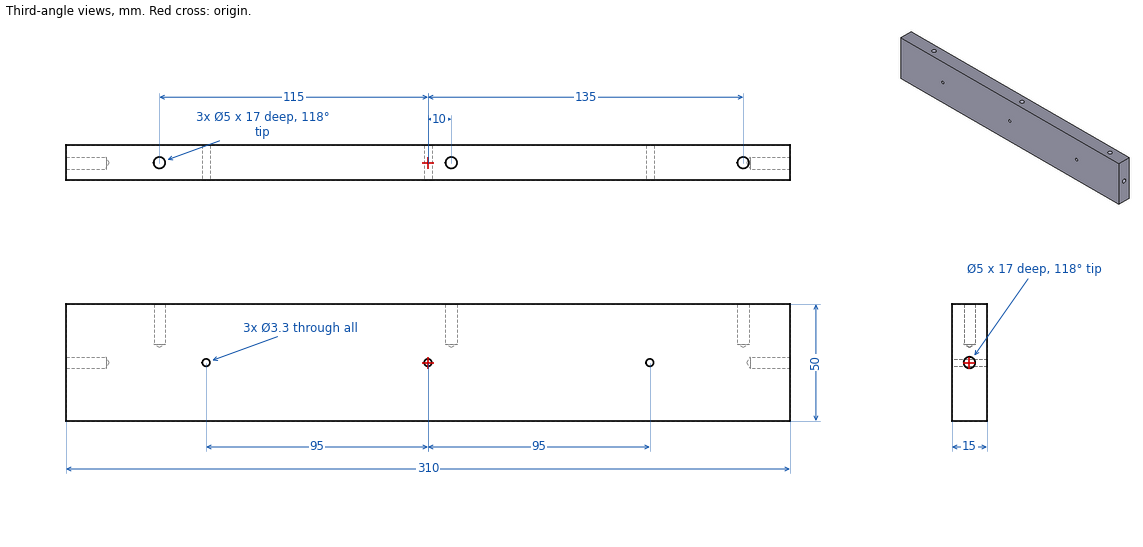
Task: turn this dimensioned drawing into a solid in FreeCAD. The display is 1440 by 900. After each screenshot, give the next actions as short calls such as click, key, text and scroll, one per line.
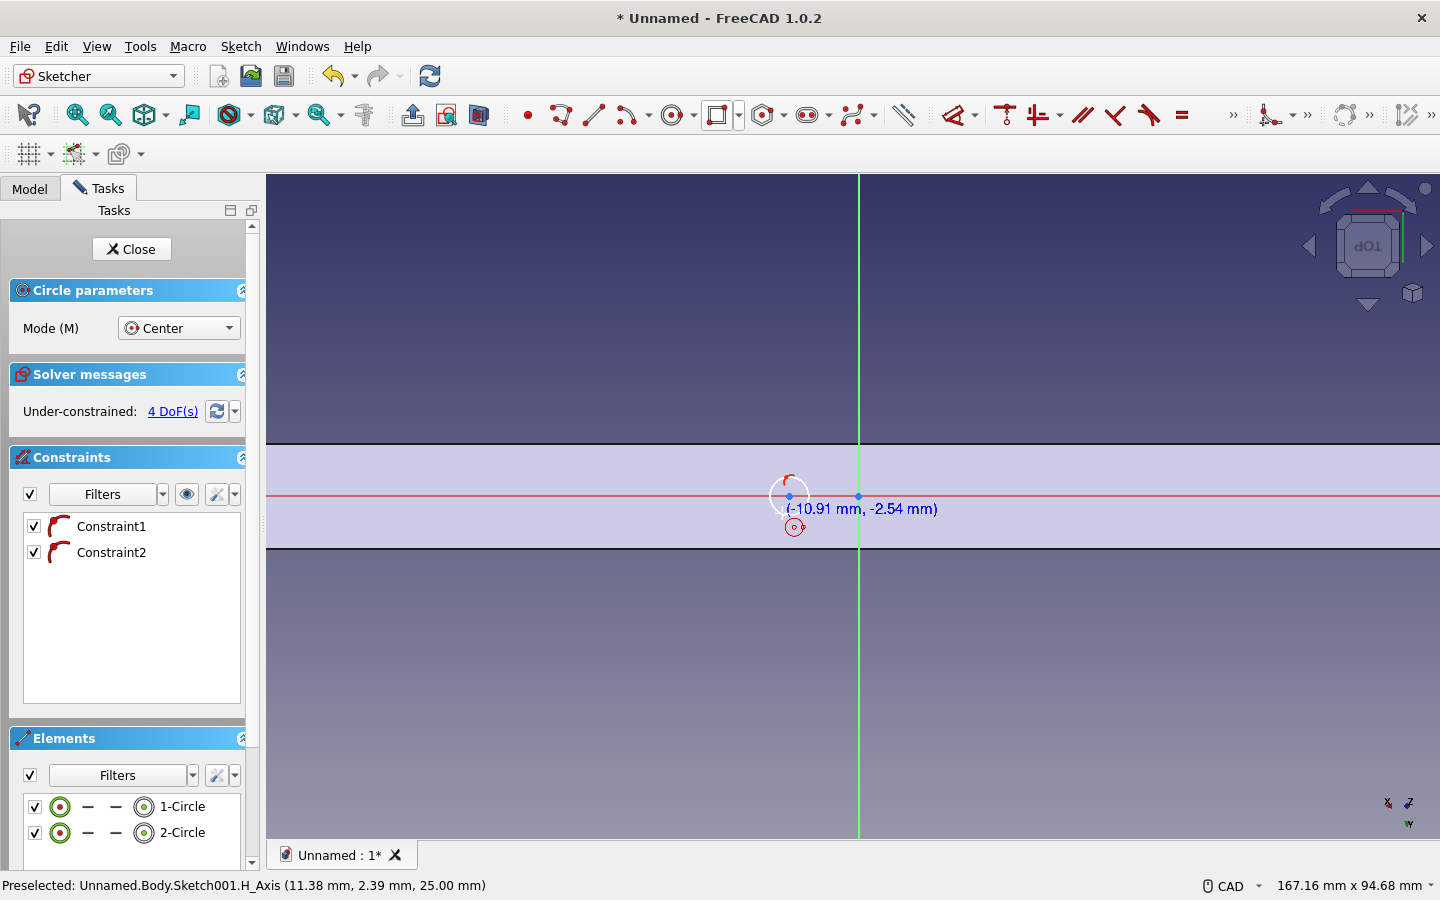
scroll(782, 513, down, 5)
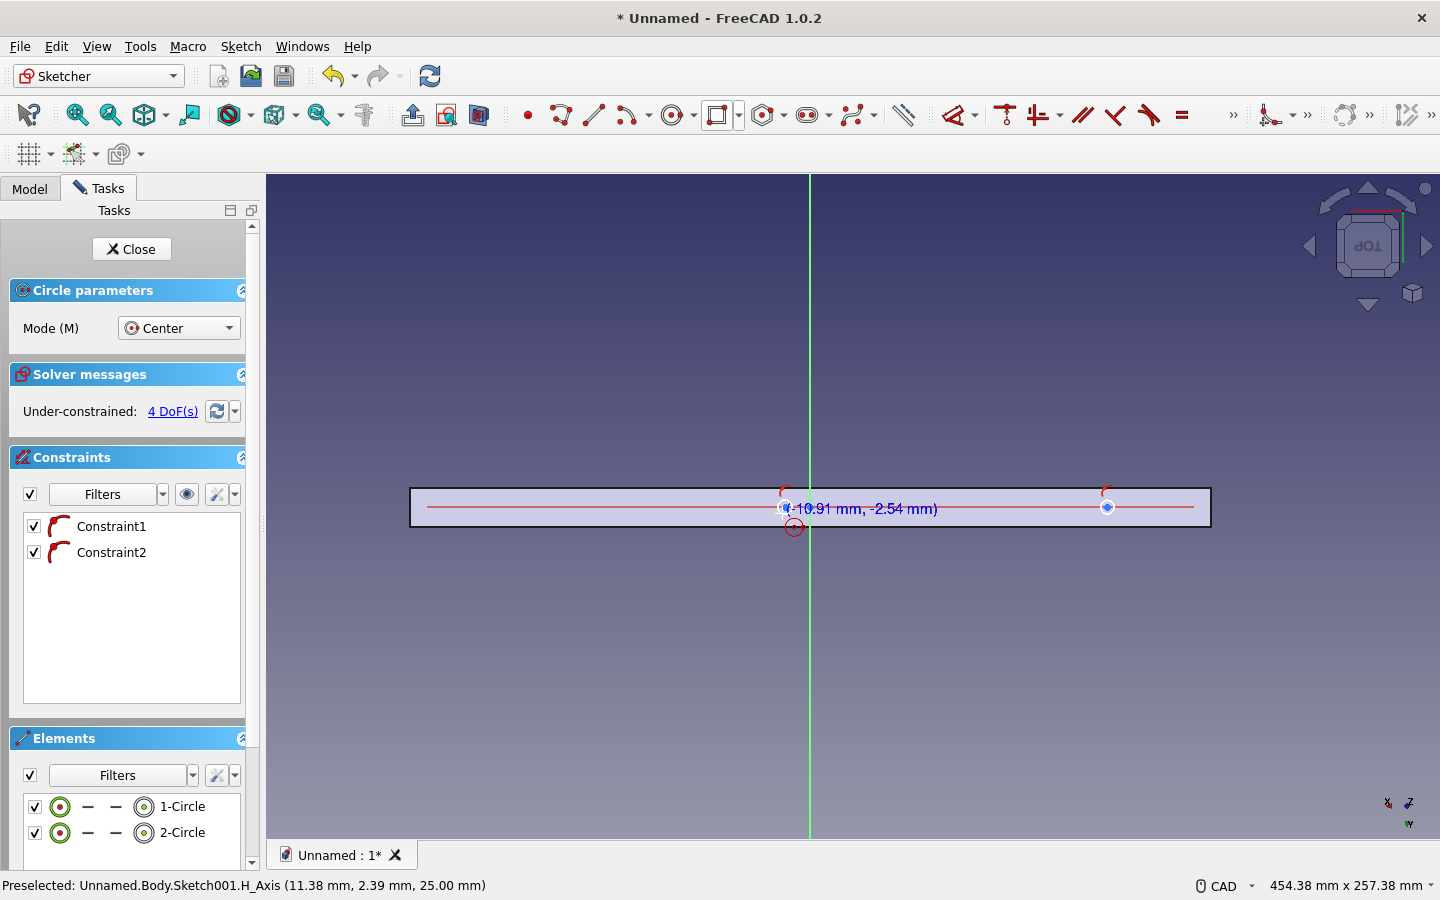
scroll(462, 507, up, 7)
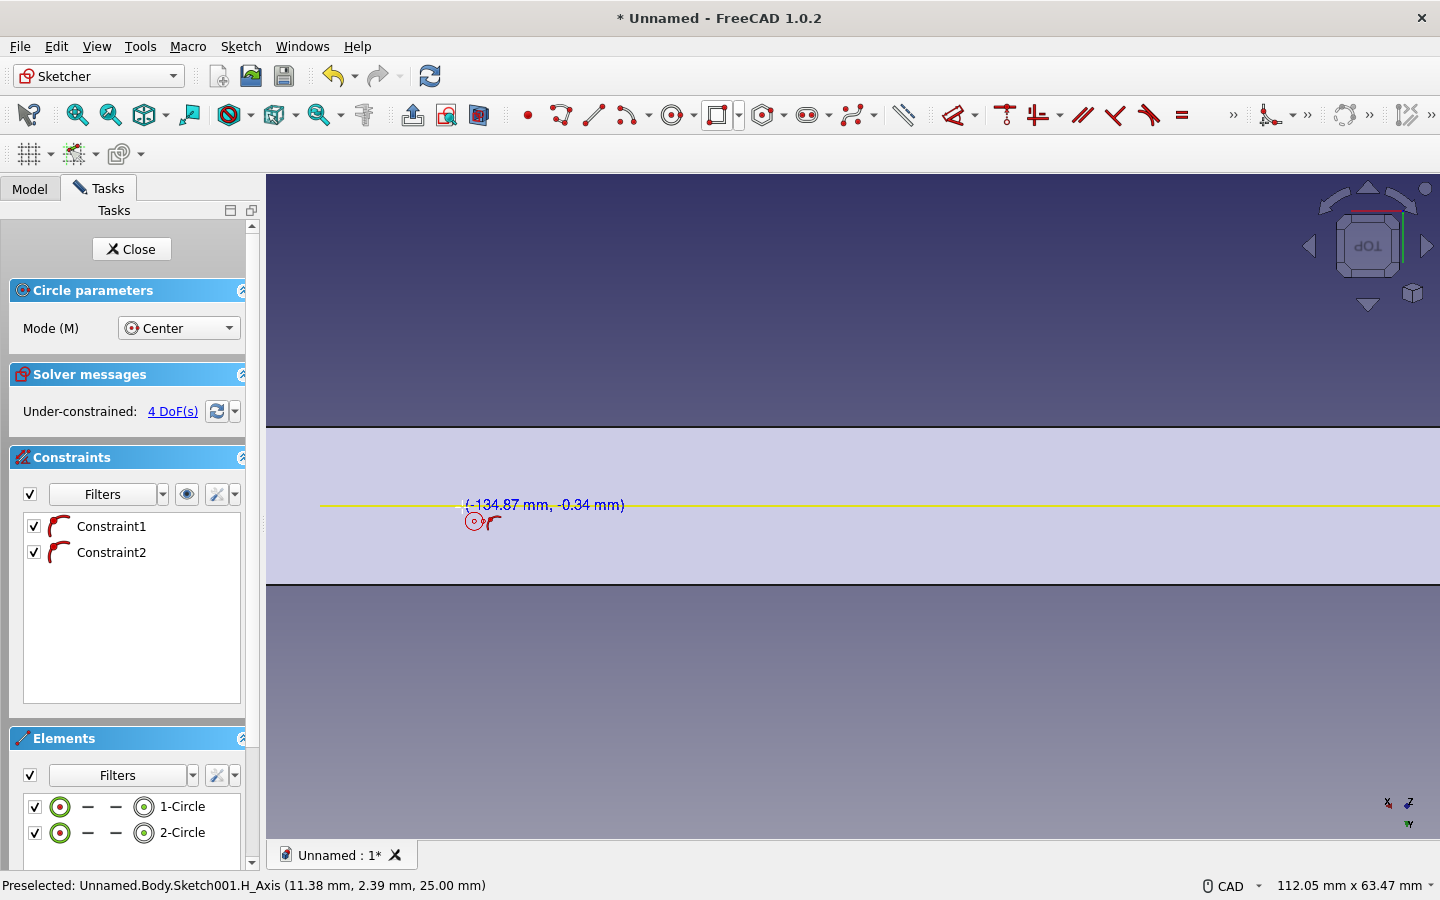
scroll(462, 507, down, 7)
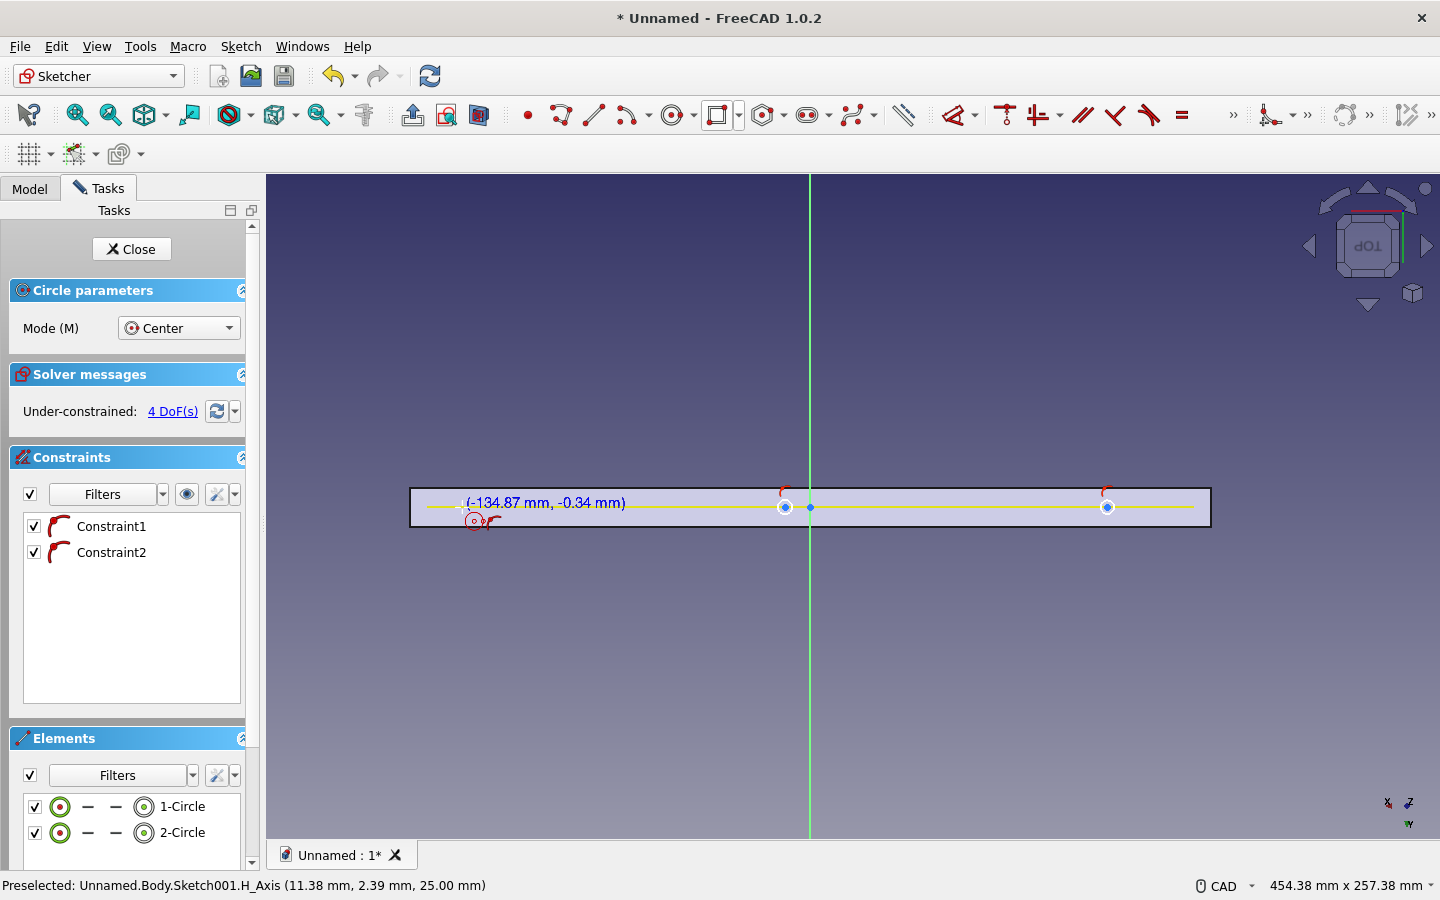
click(462, 507)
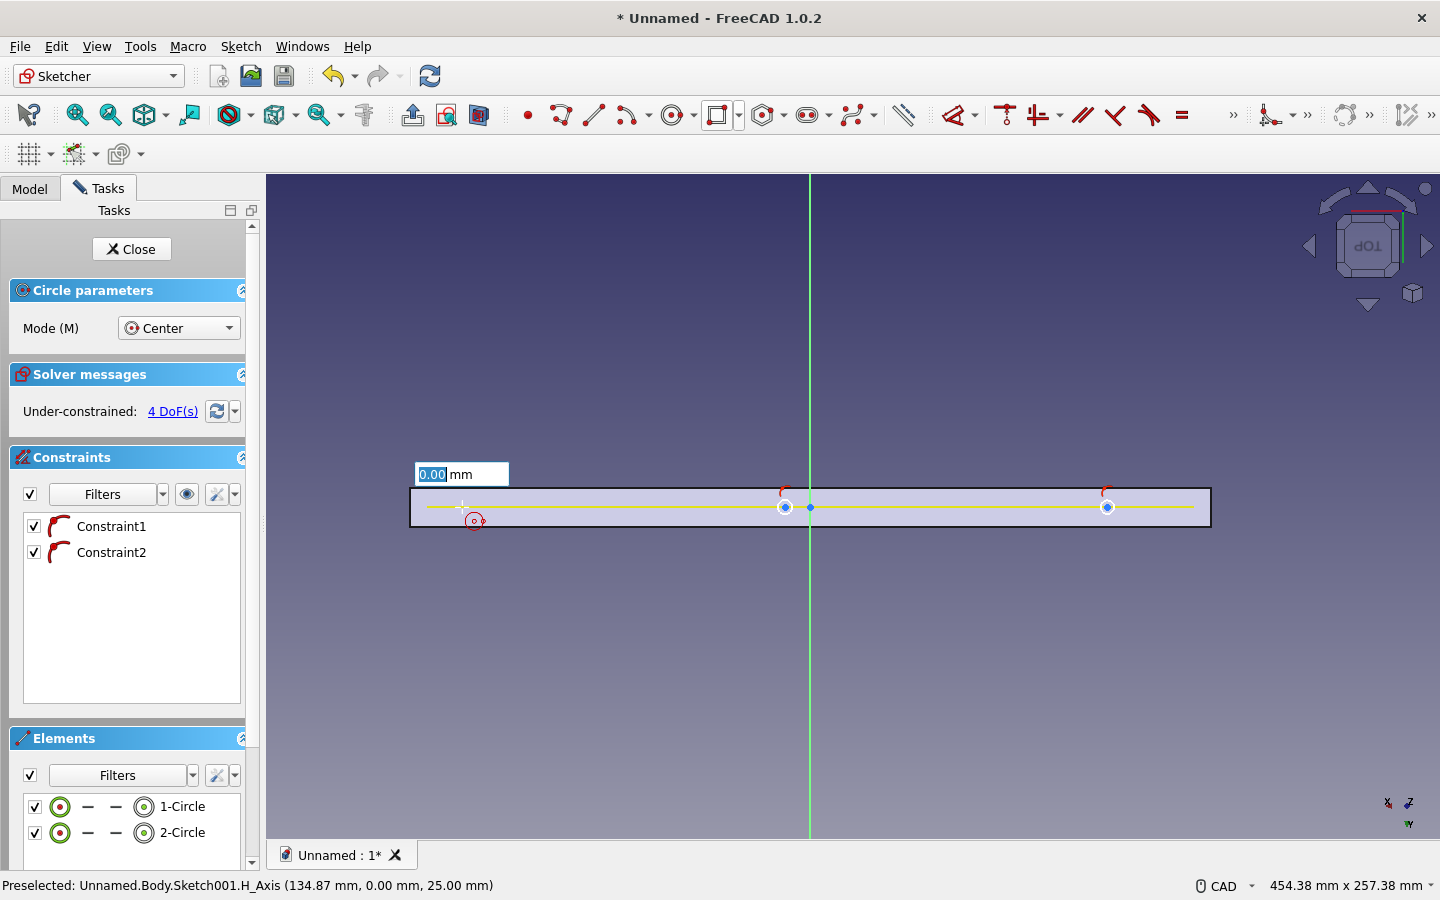
scroll(459, 513, up, 5)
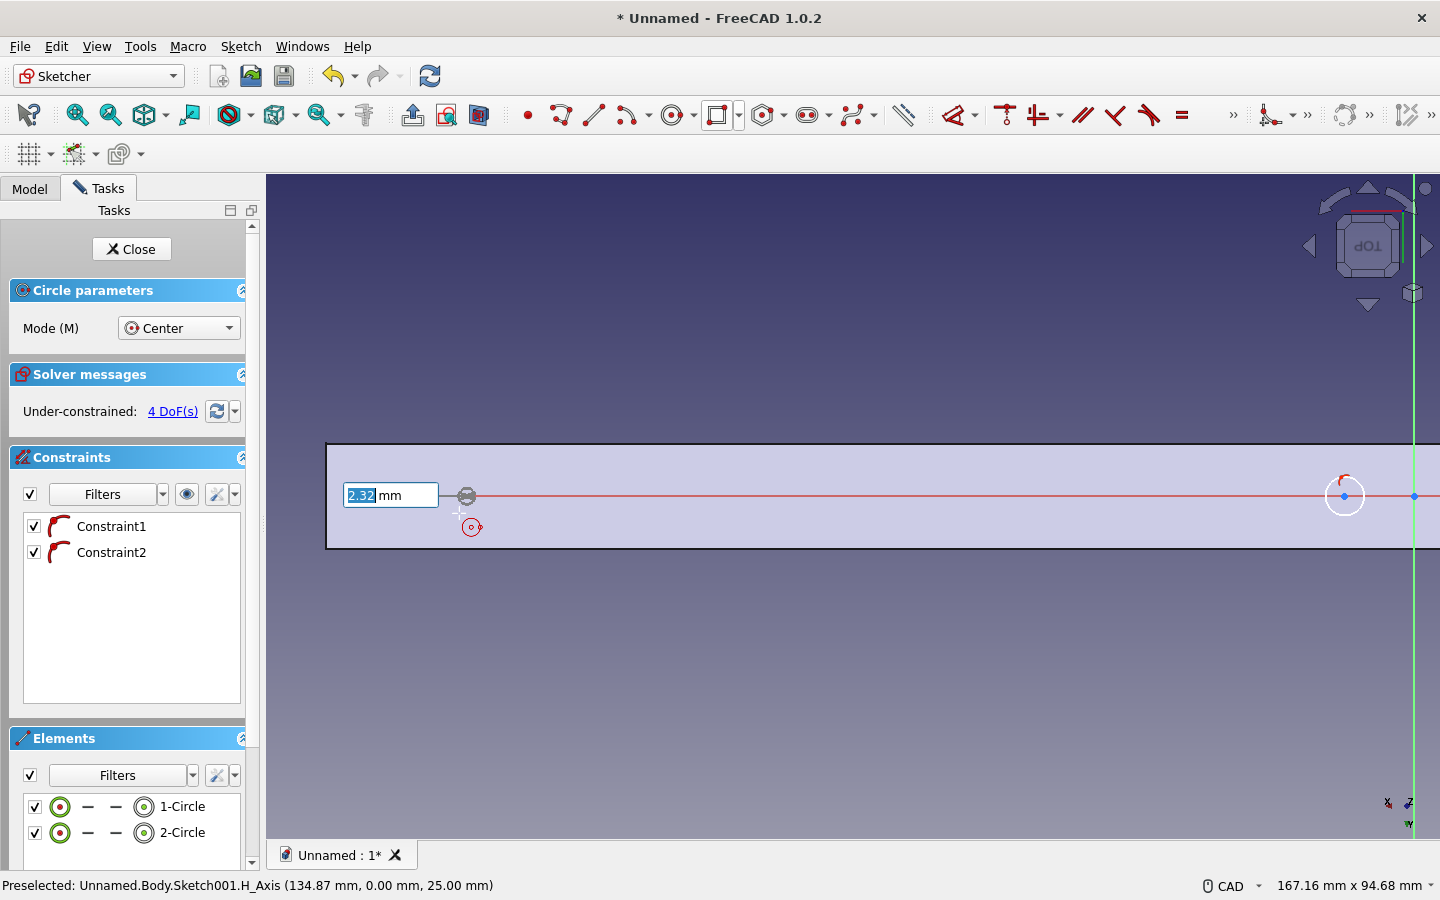
click(460, 513)
key(Escape)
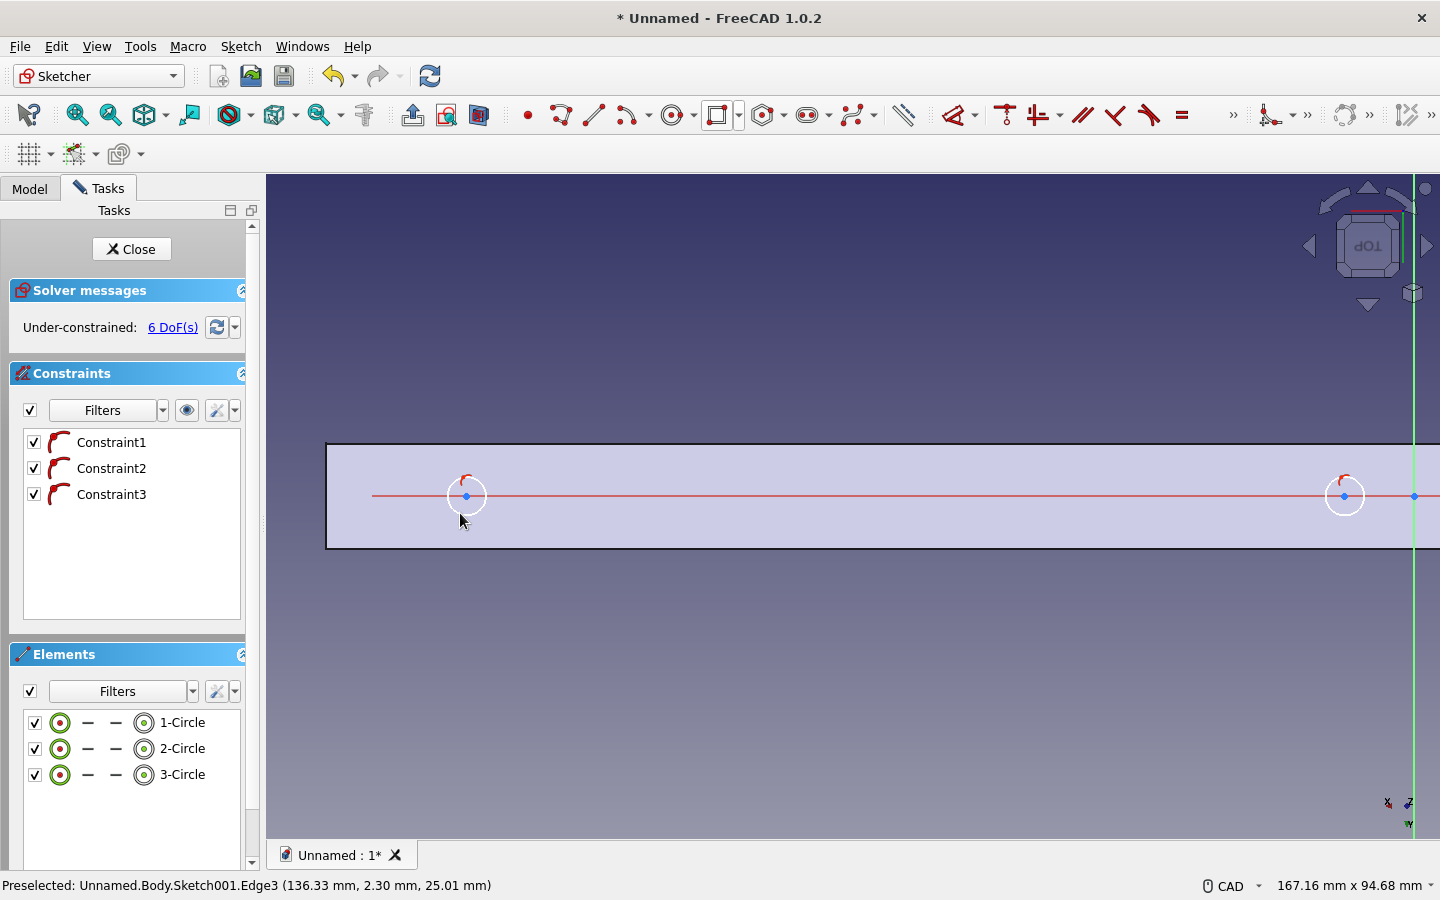
scroll(459, 513, down, 5)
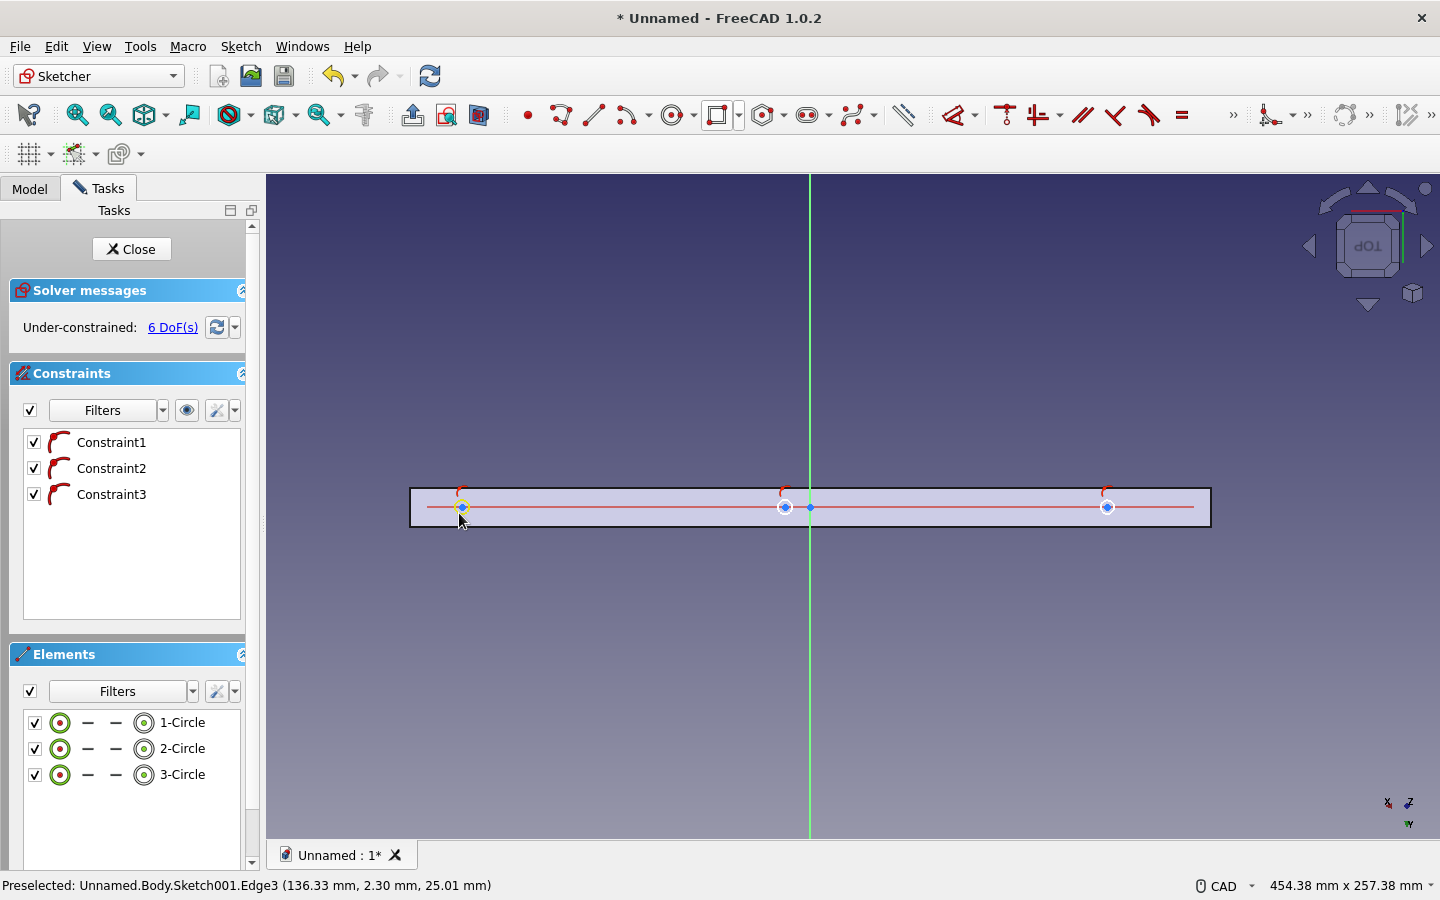
scroll(1112, 502, up, 6)